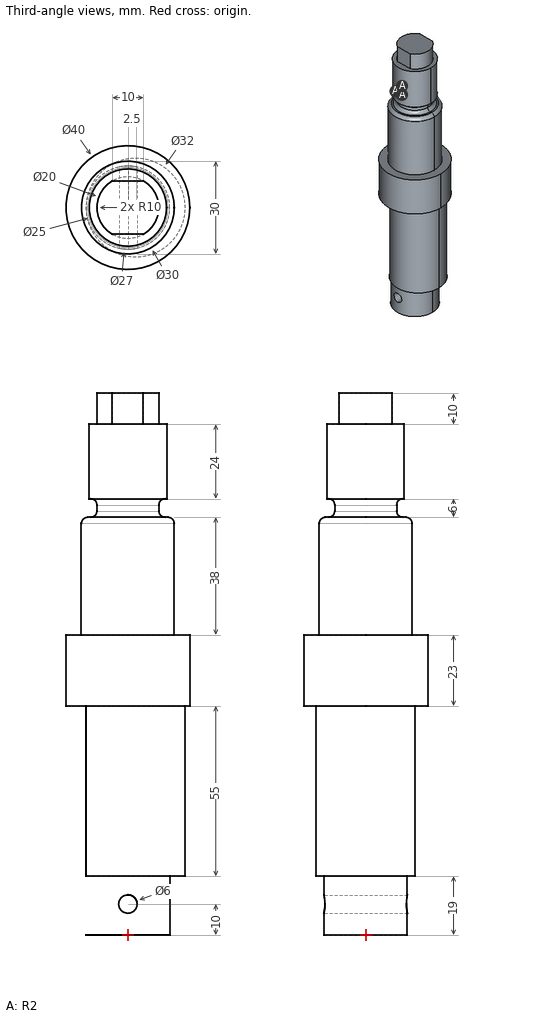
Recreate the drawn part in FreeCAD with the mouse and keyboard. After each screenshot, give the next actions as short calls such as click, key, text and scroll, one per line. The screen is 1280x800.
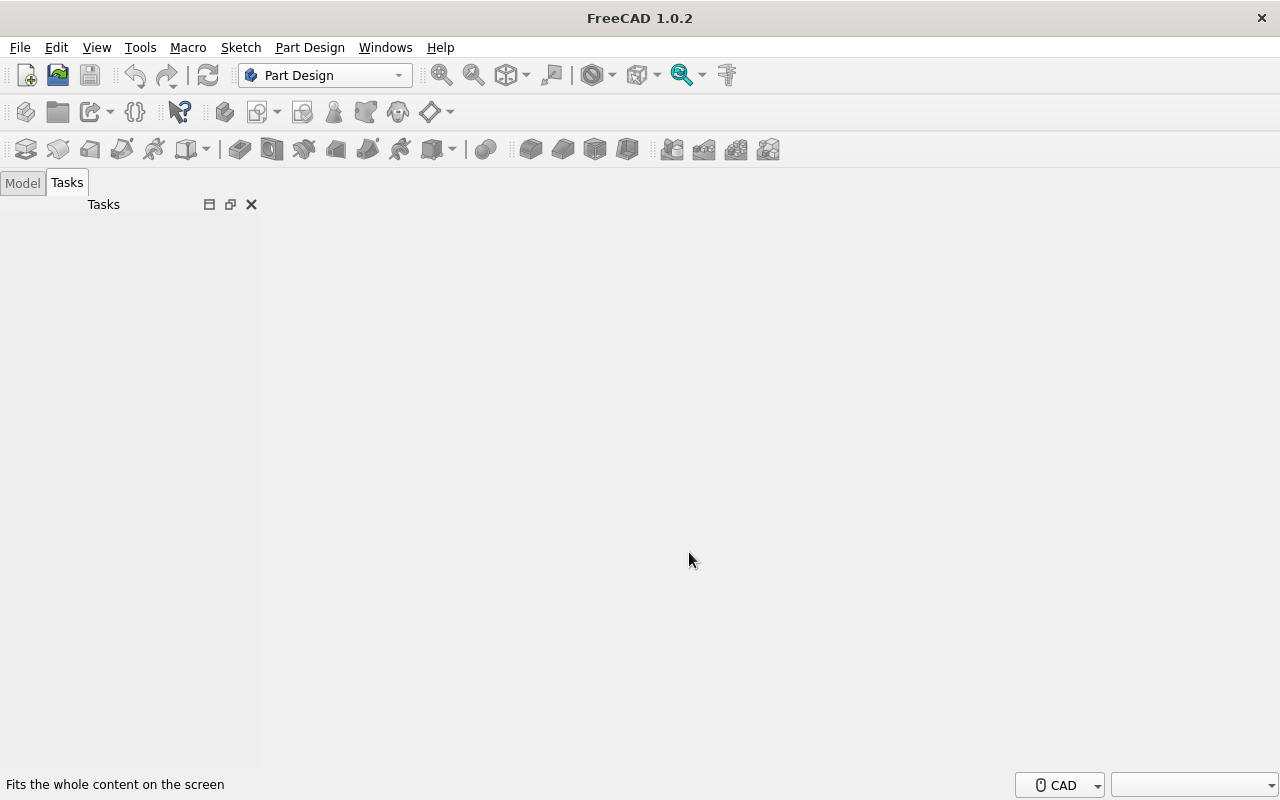
key(ctrl+n)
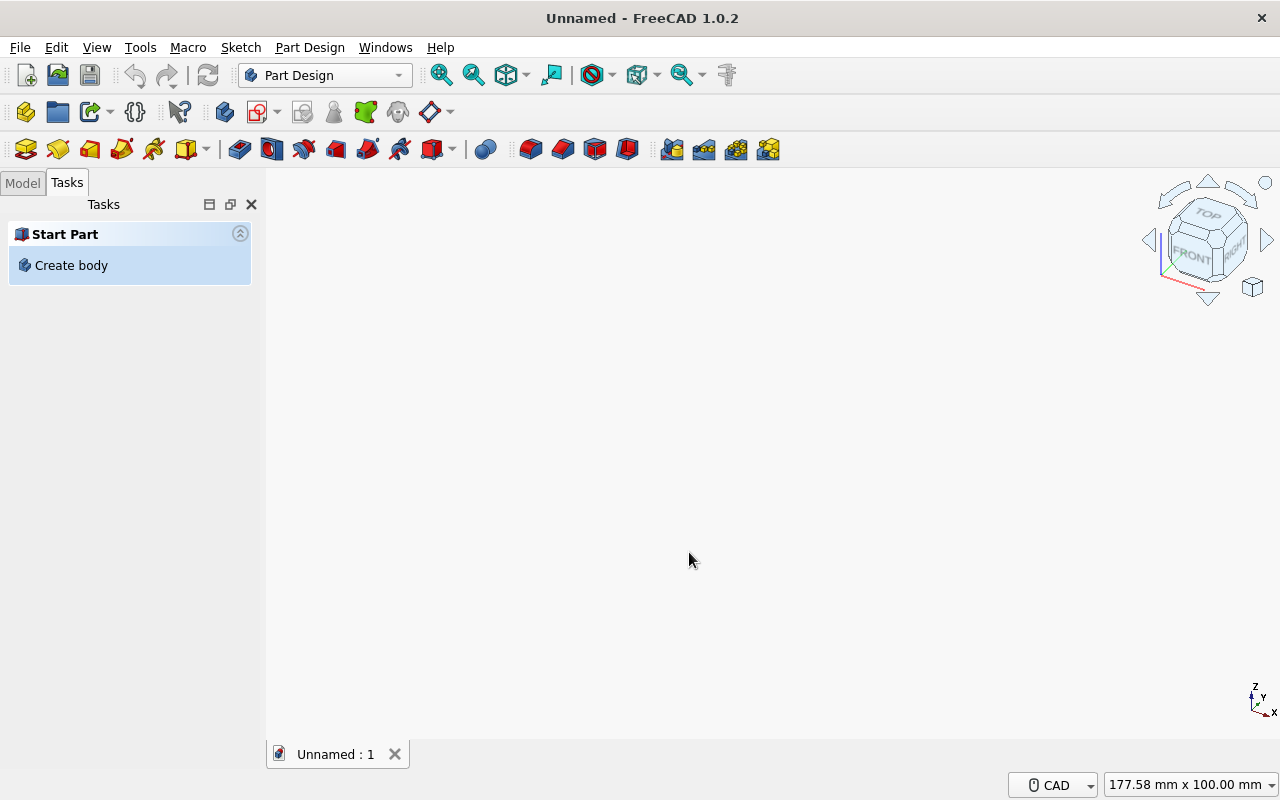
click(258, 112)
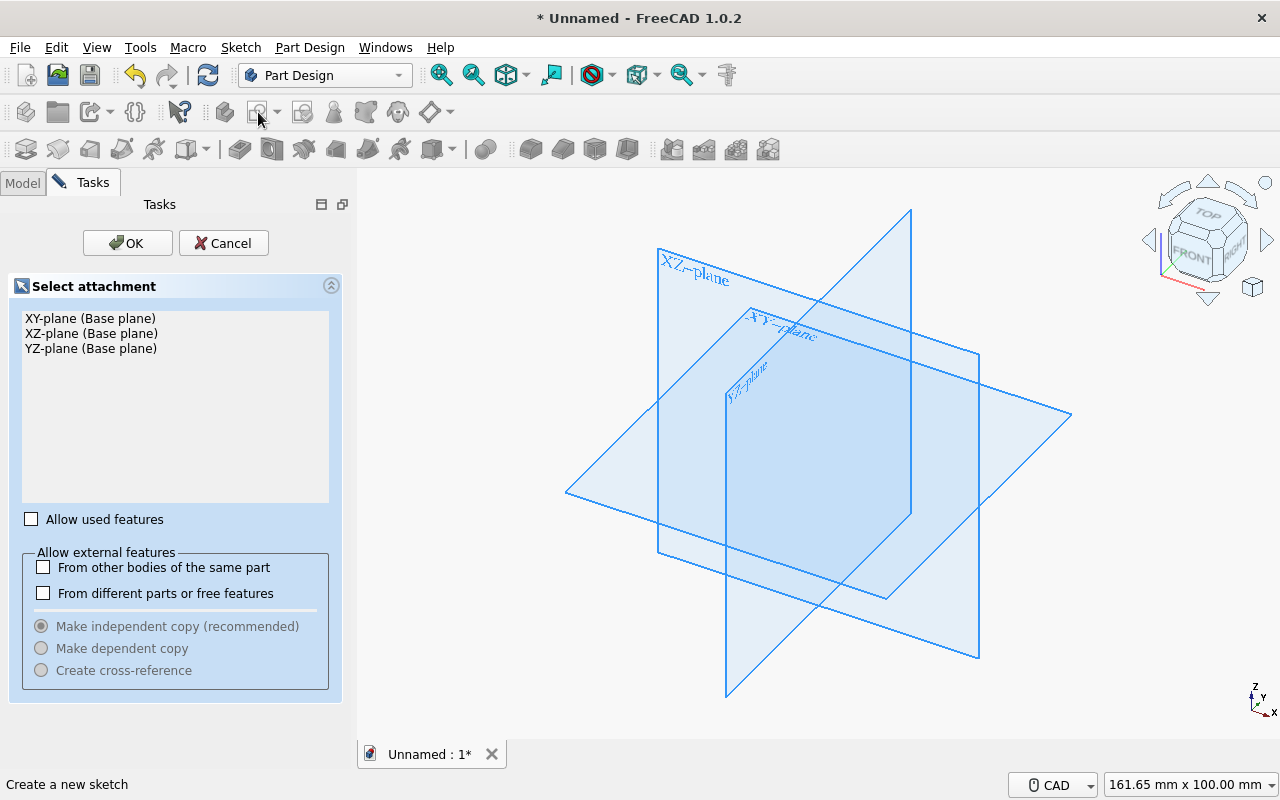
click(82, 318)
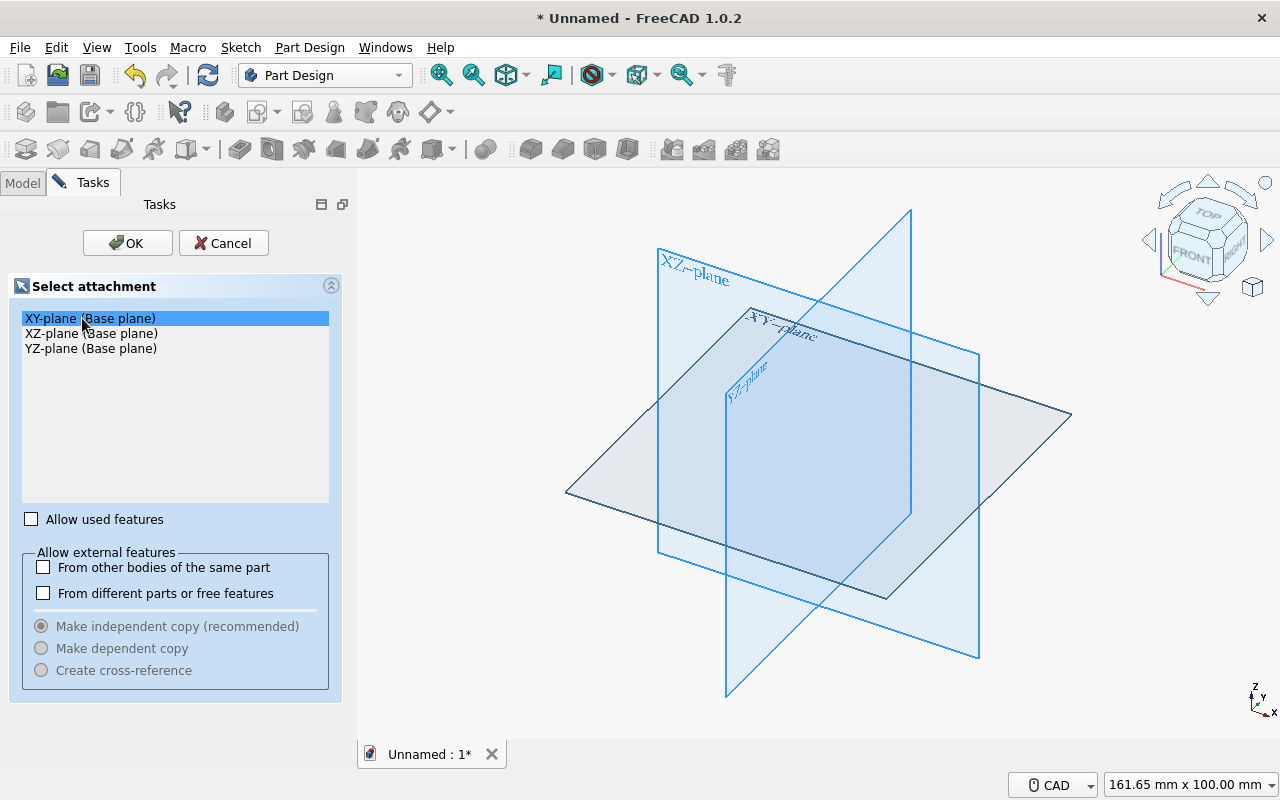
click(128, 243)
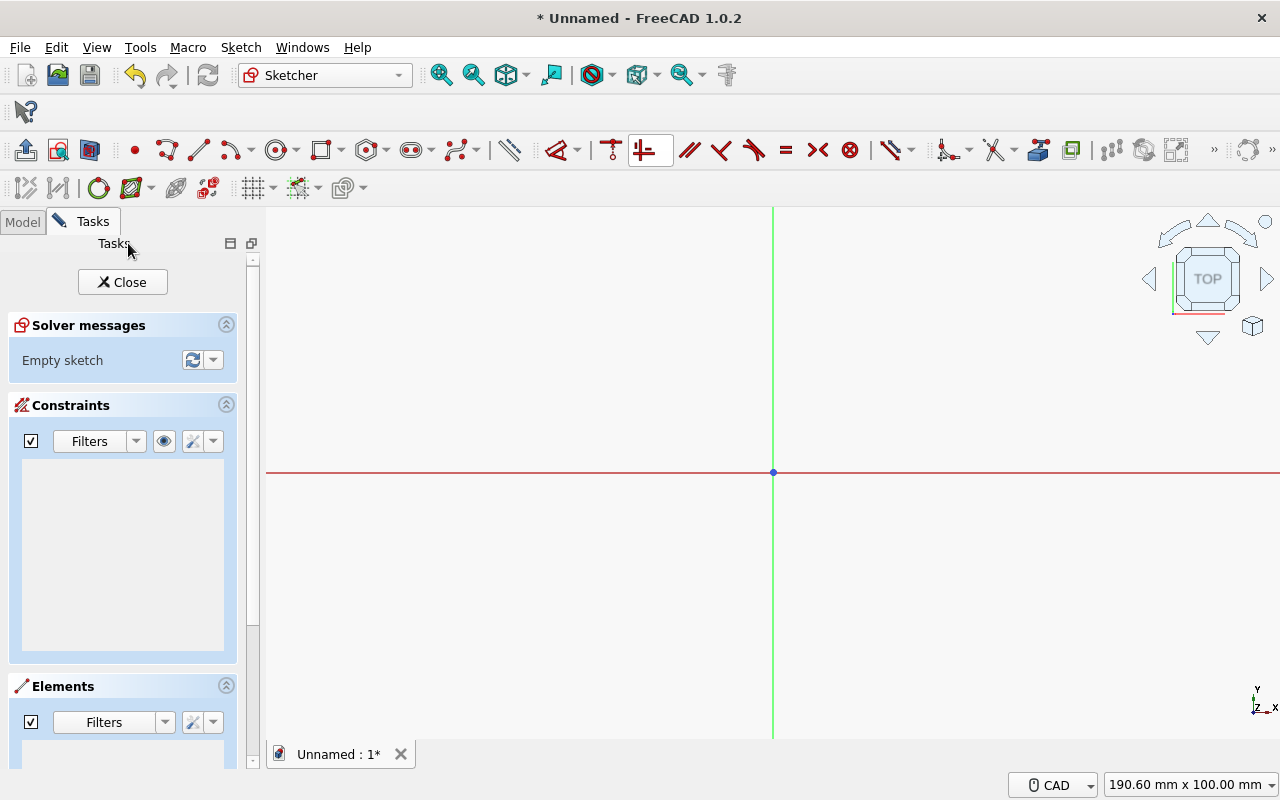
scroll(829, 473, up, 4)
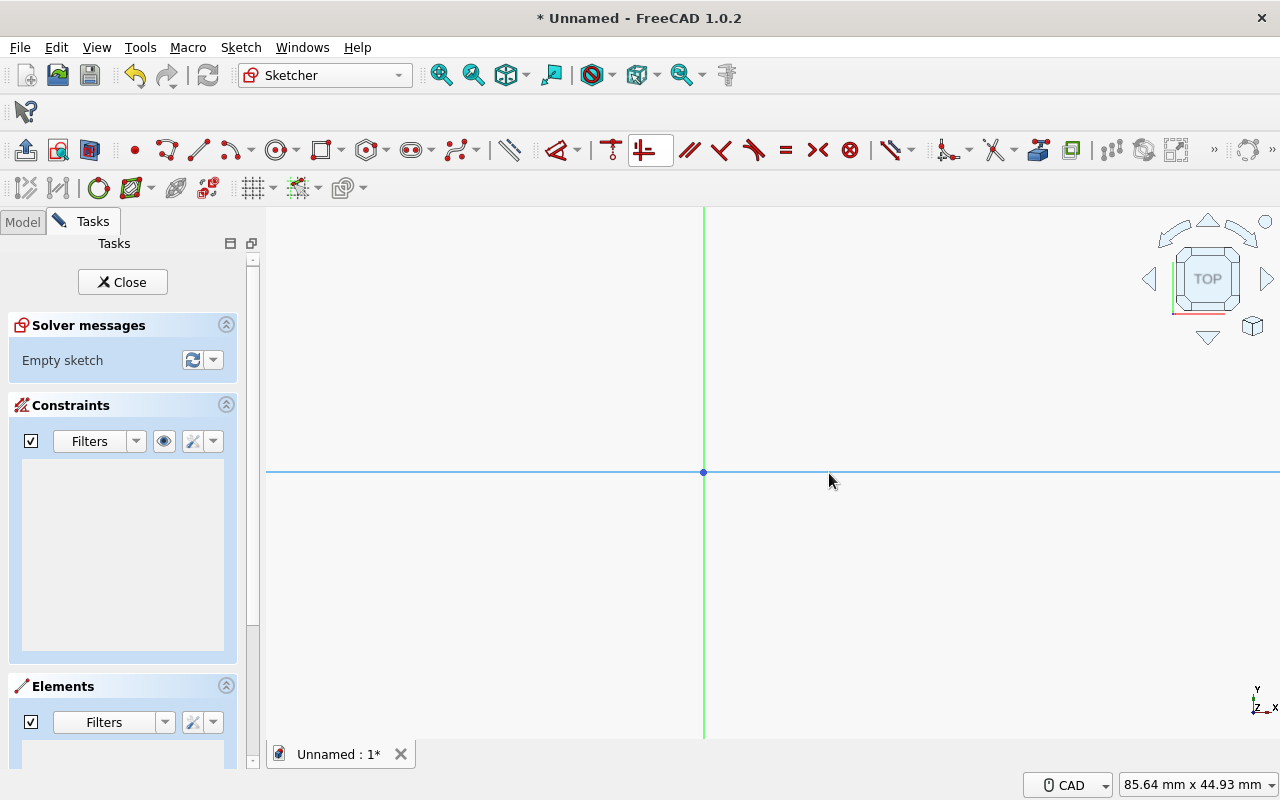
key(g)
key(c)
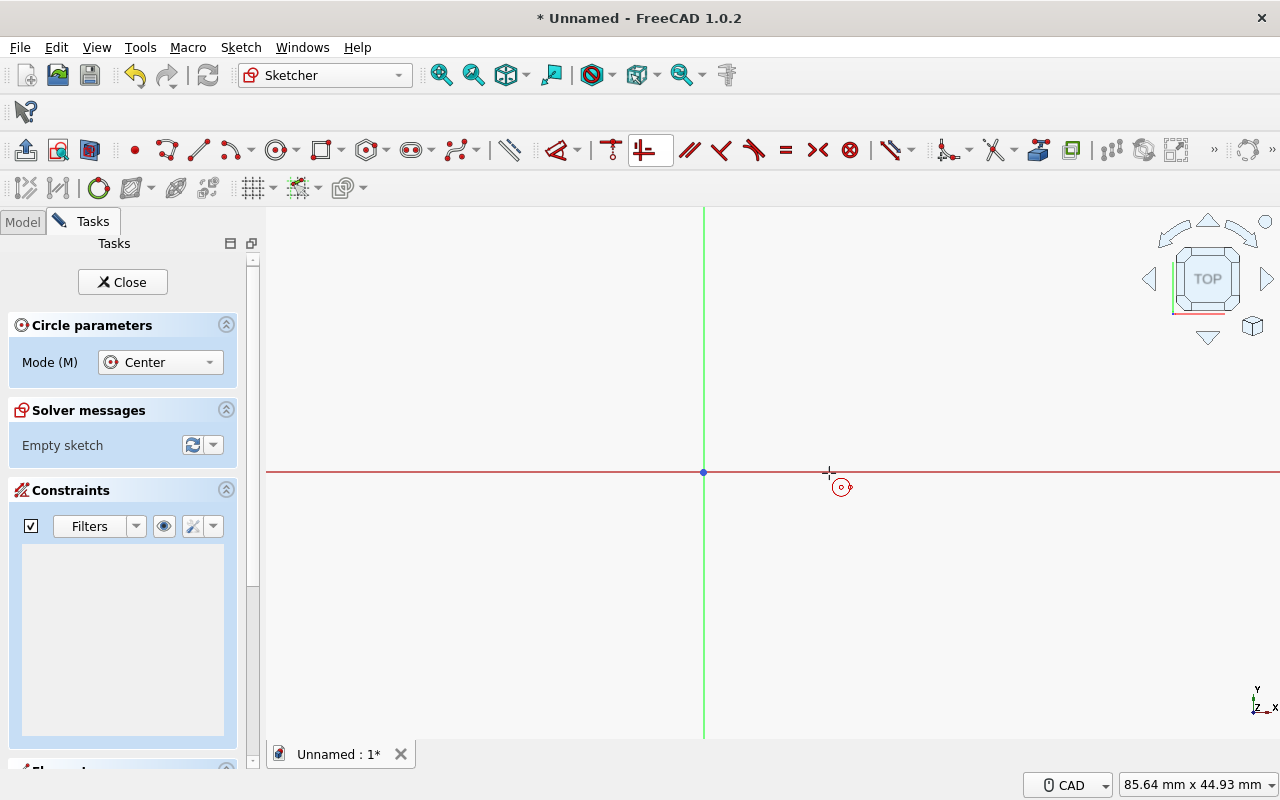
click(704, 472)
click(817, 359)
key(Escape)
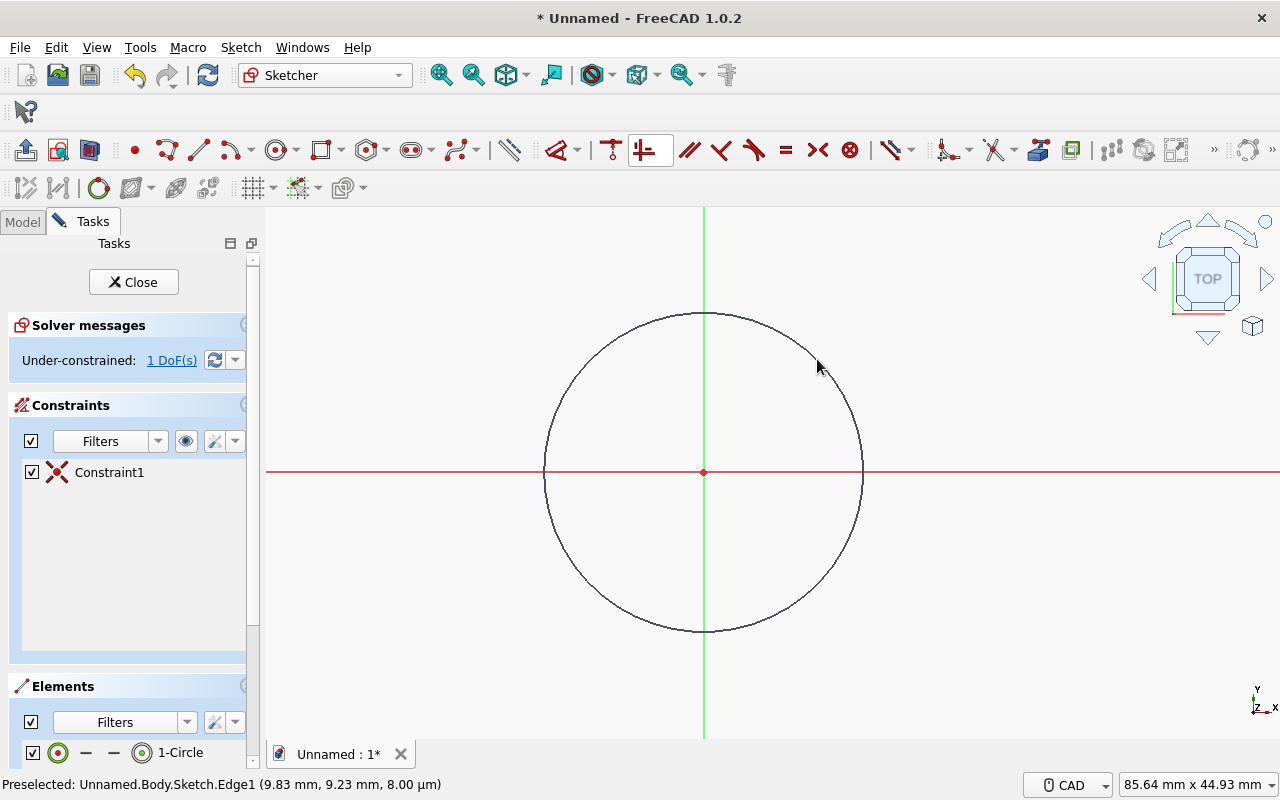
click(556, 150)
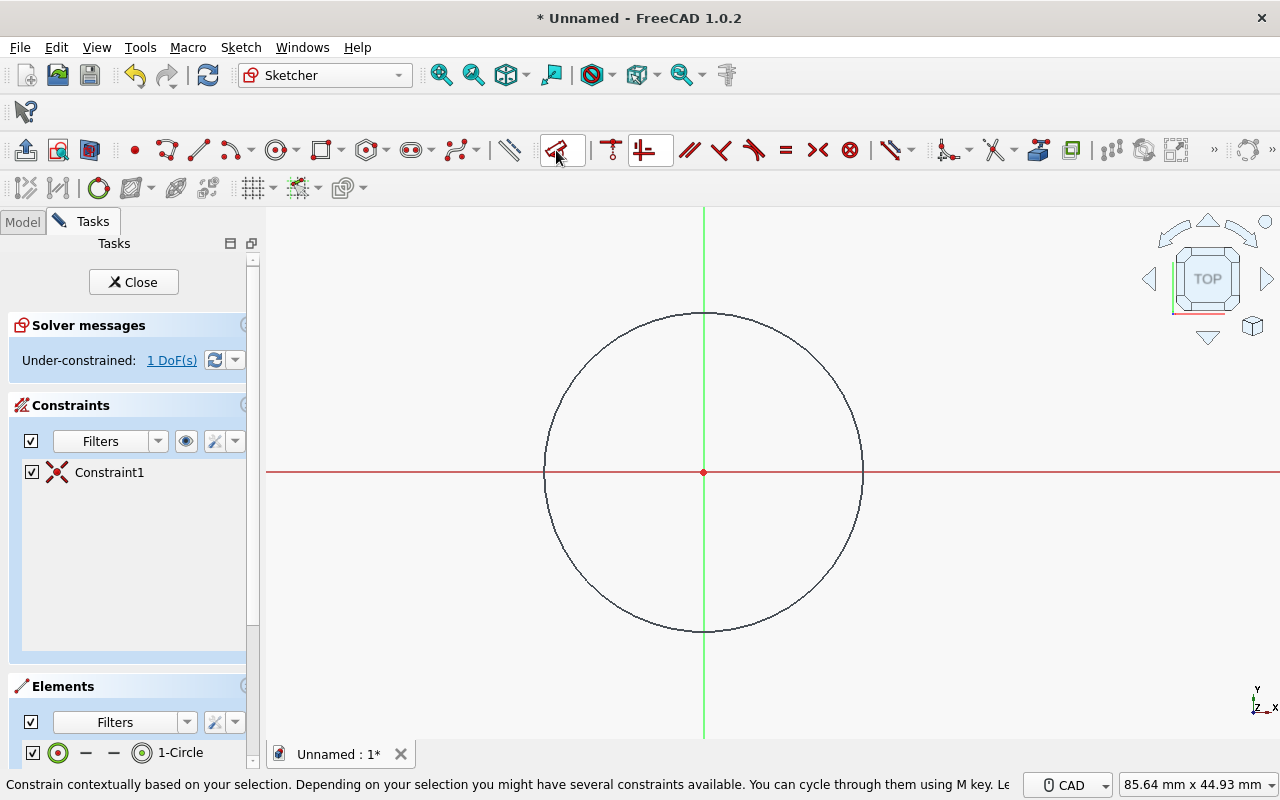
click(816, 359)
click(839, 336)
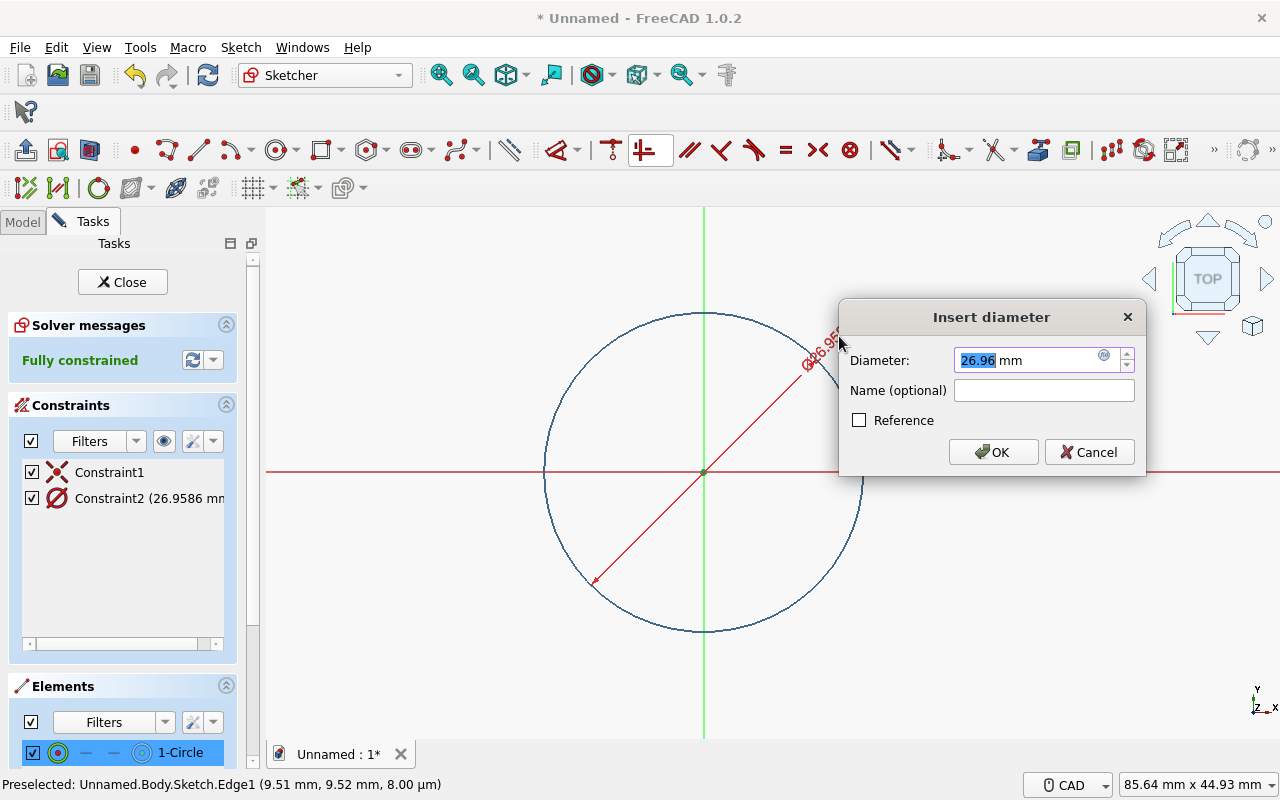
text(27)
key(Return)
key(Escape)